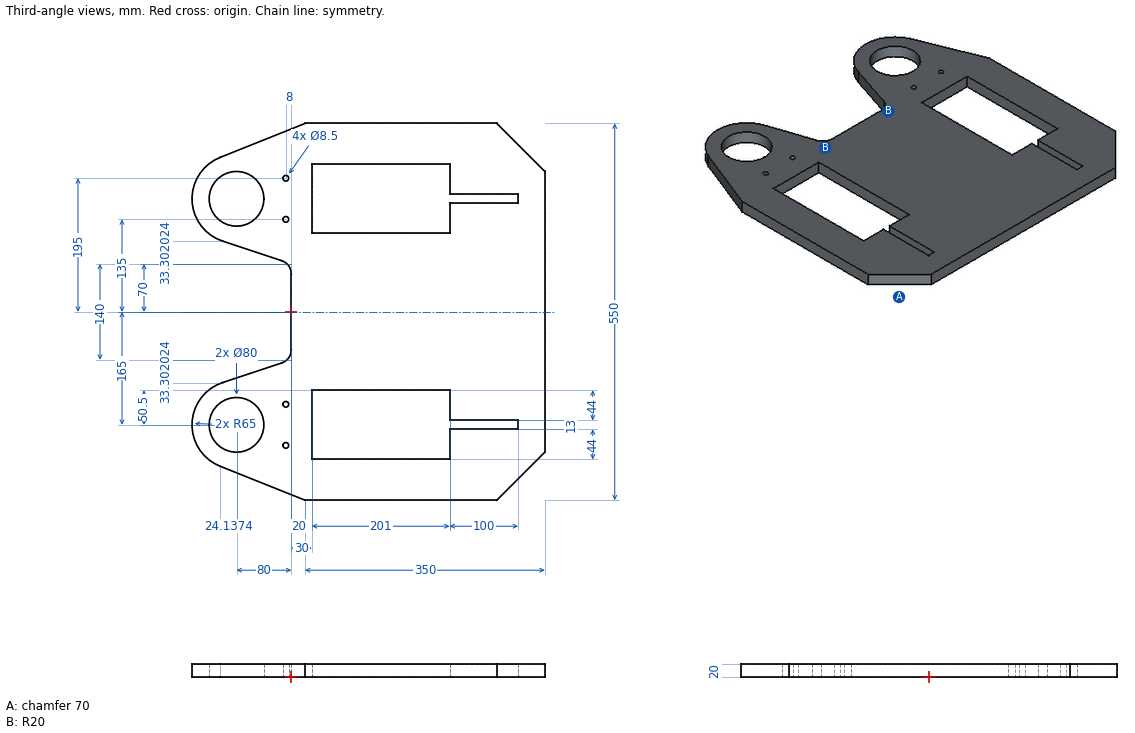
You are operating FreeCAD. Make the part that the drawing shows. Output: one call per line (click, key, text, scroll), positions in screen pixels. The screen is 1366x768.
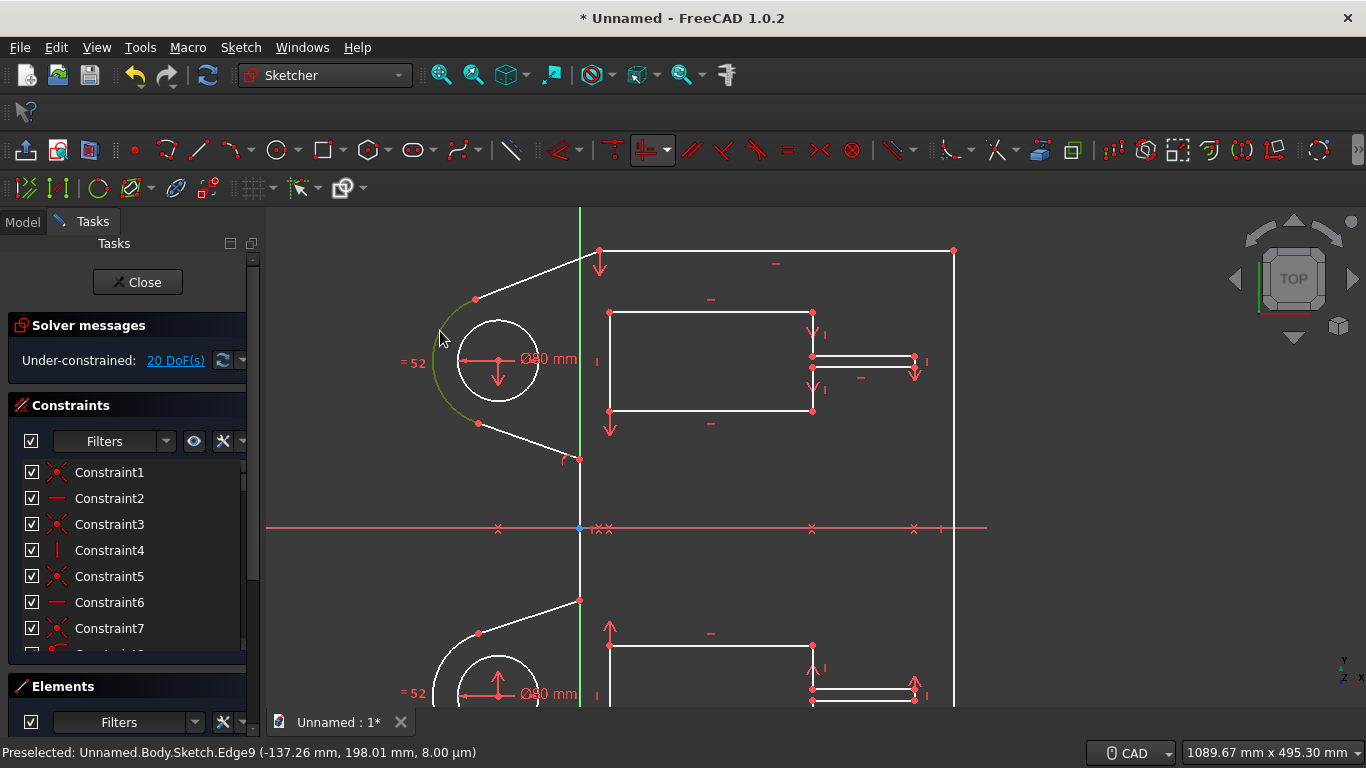
key(k)
key(r)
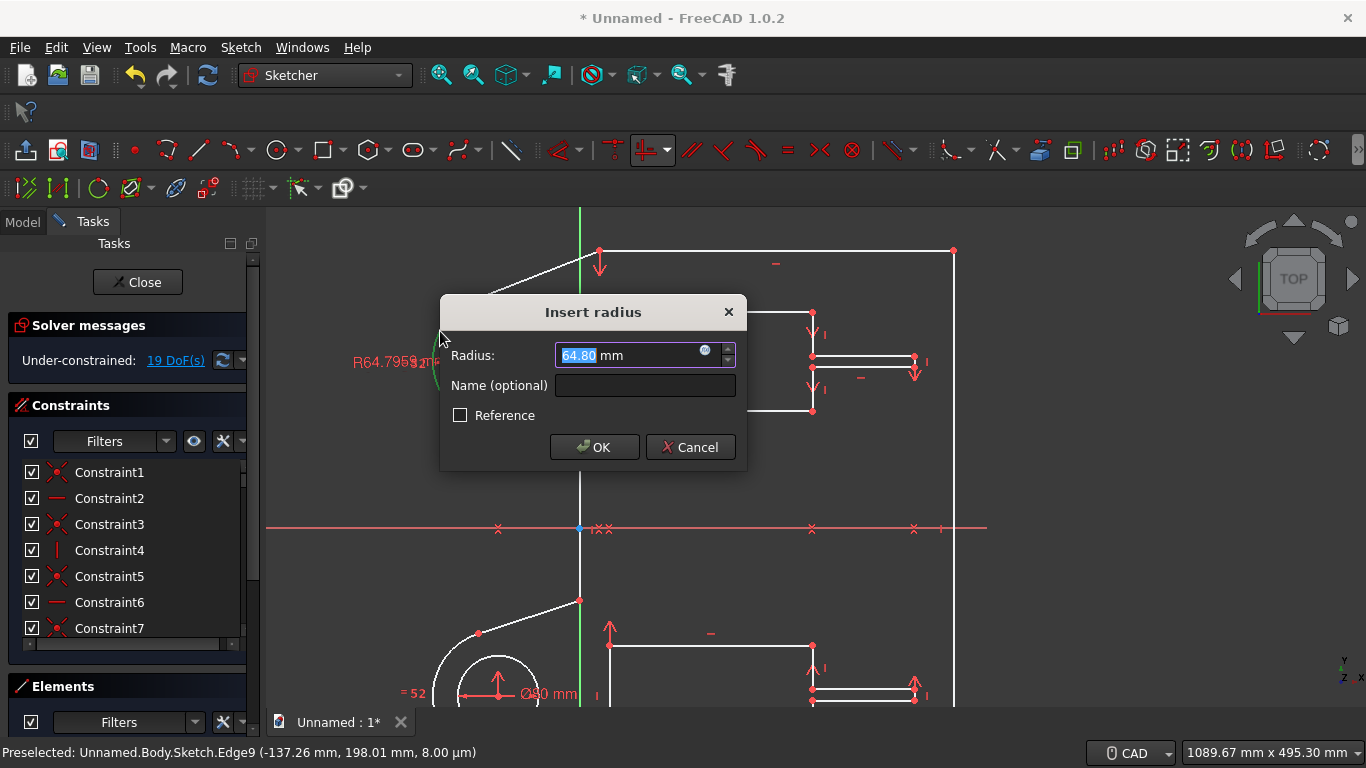
text(65)
key(Return)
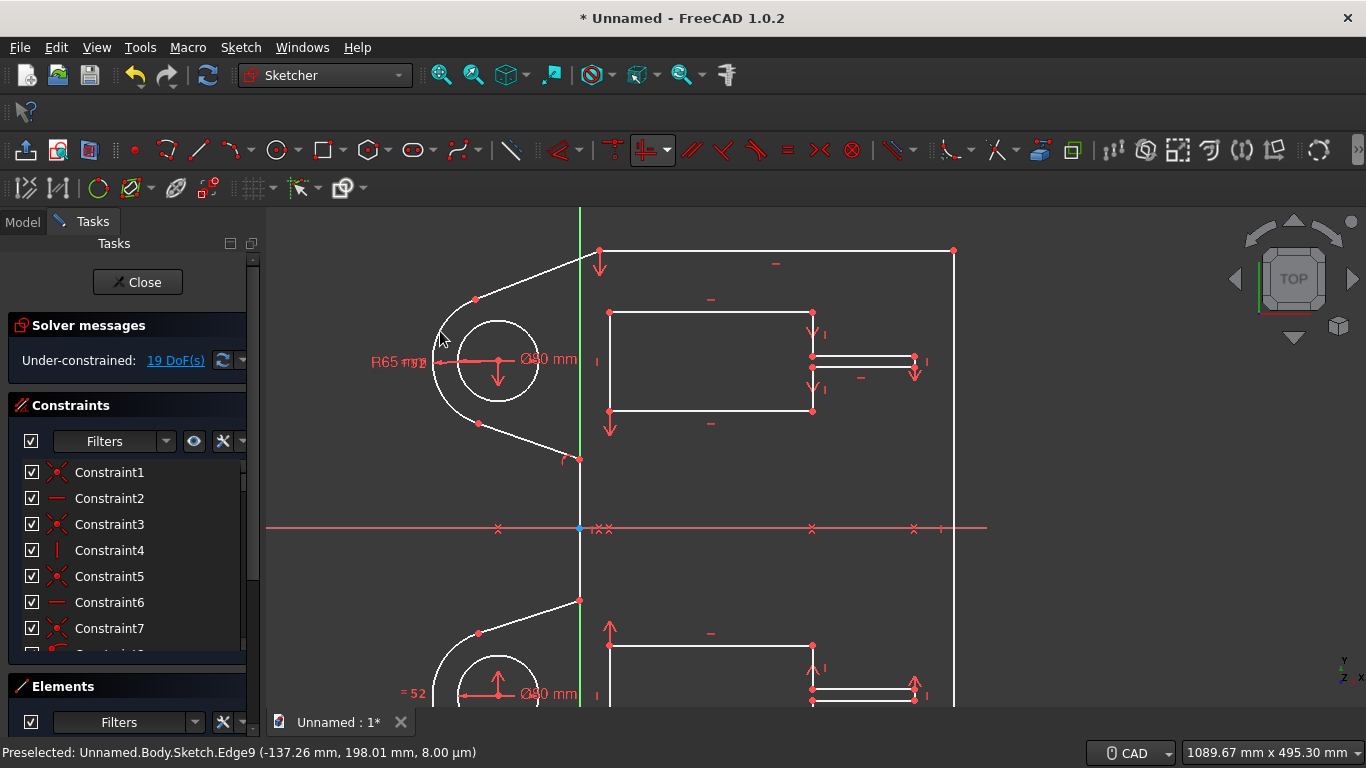
click(813, 676)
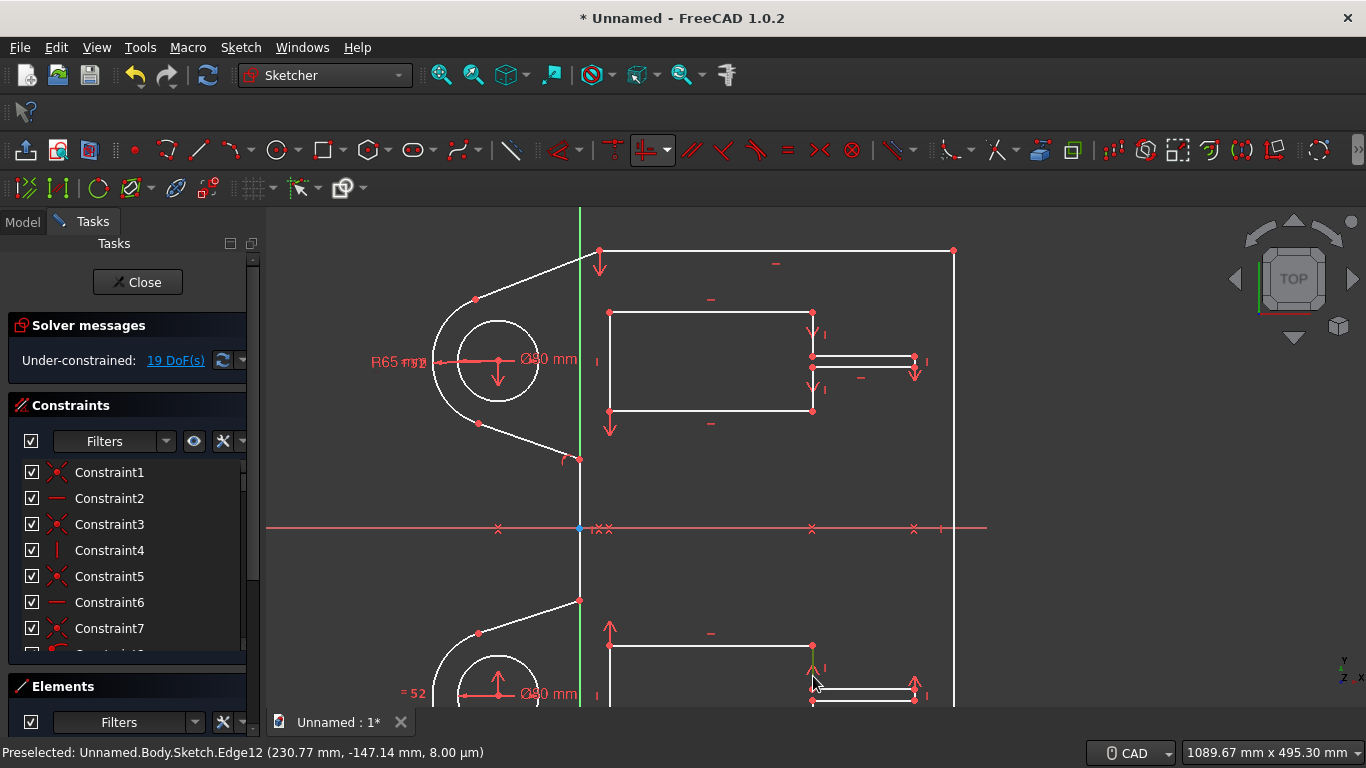
key(i)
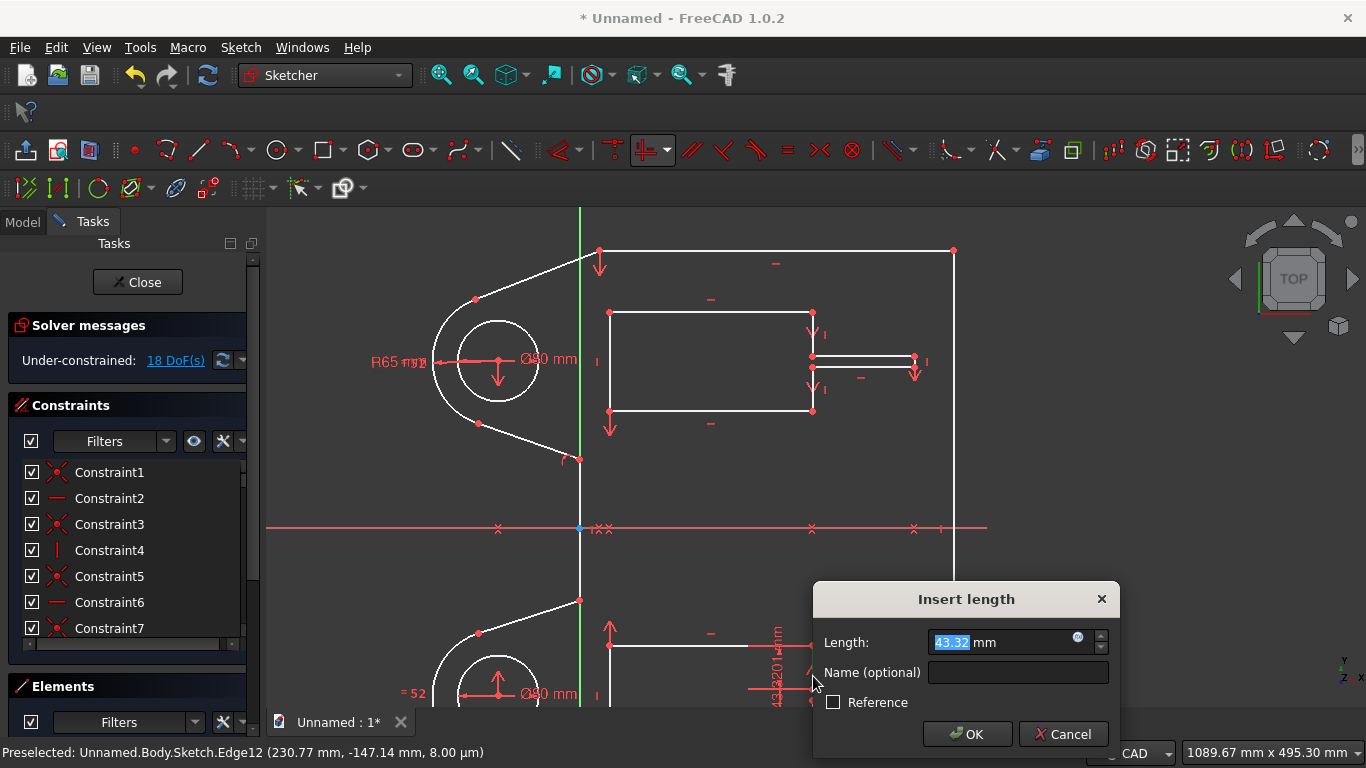
text(44)
key(Return)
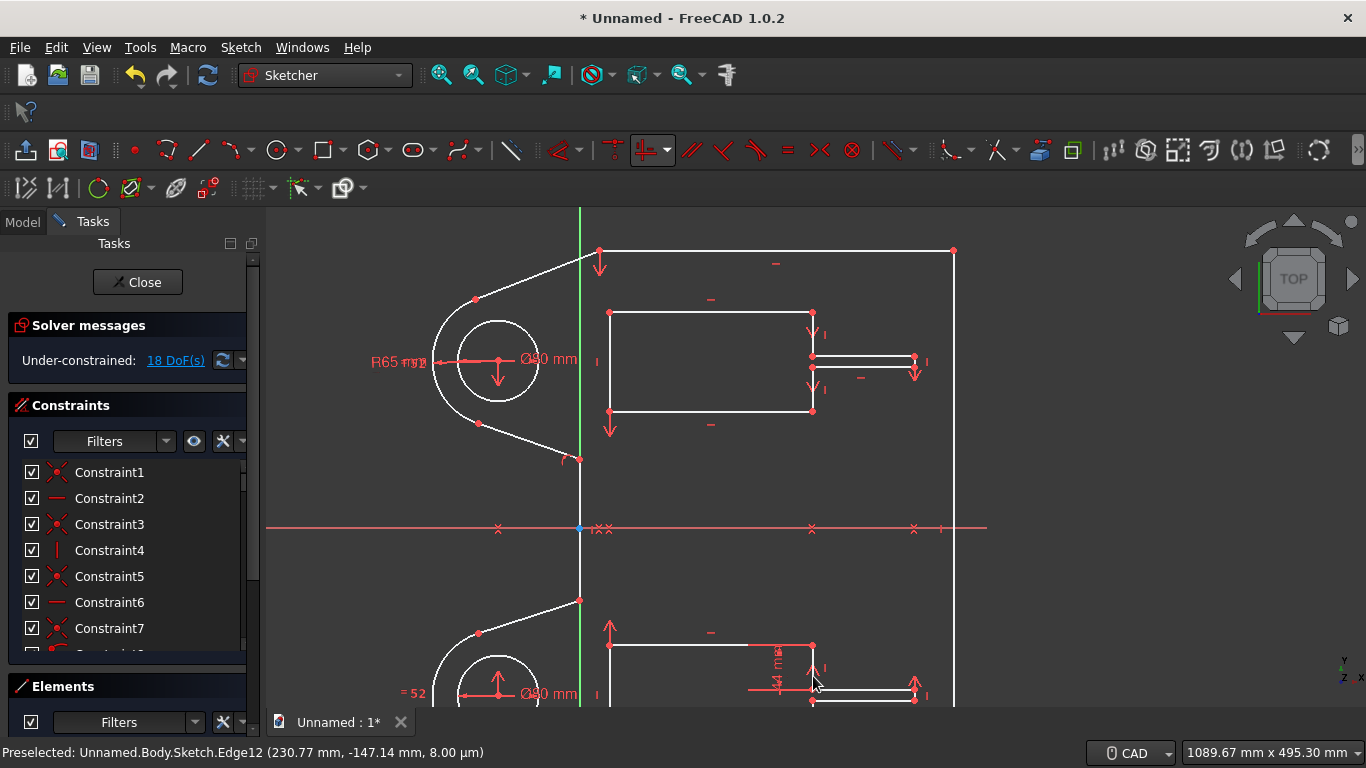
scroll(813, 370, down, 3)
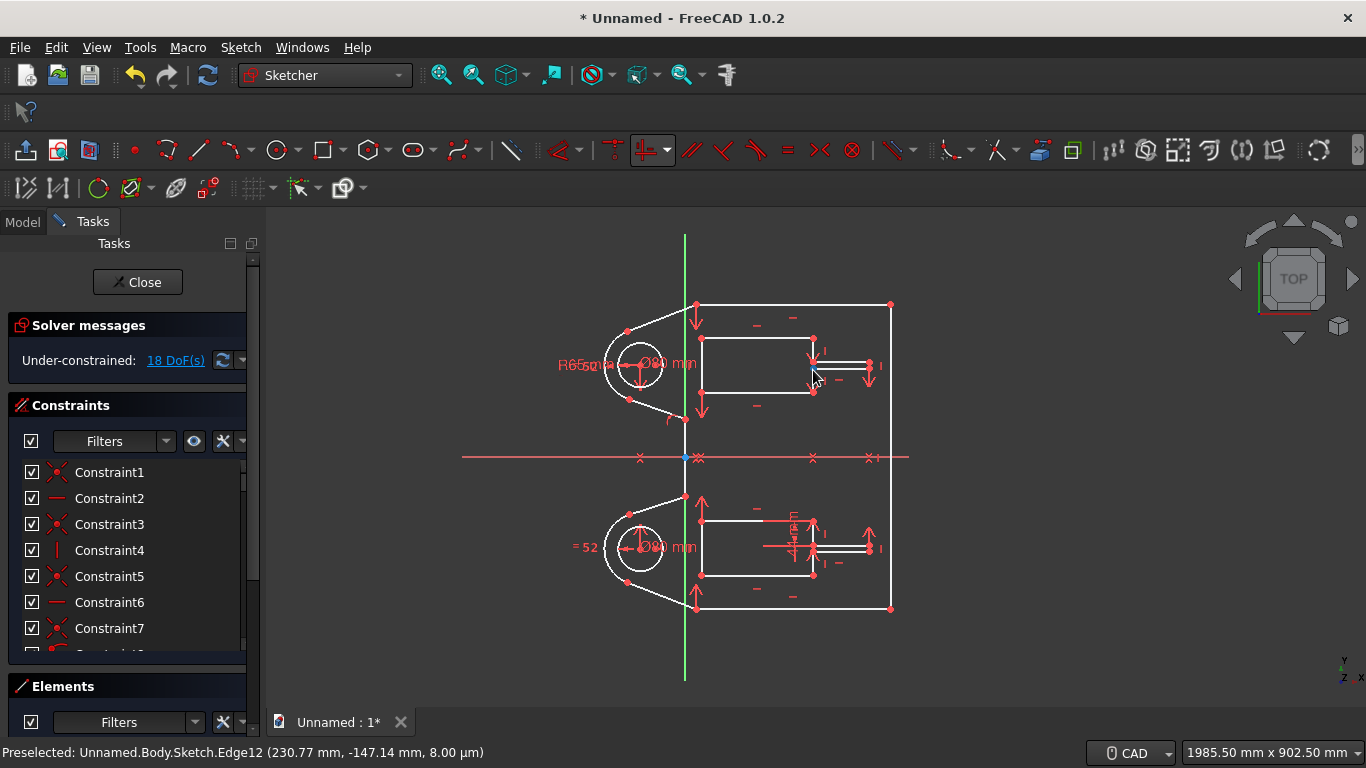
scroll(869, 549, up, 9)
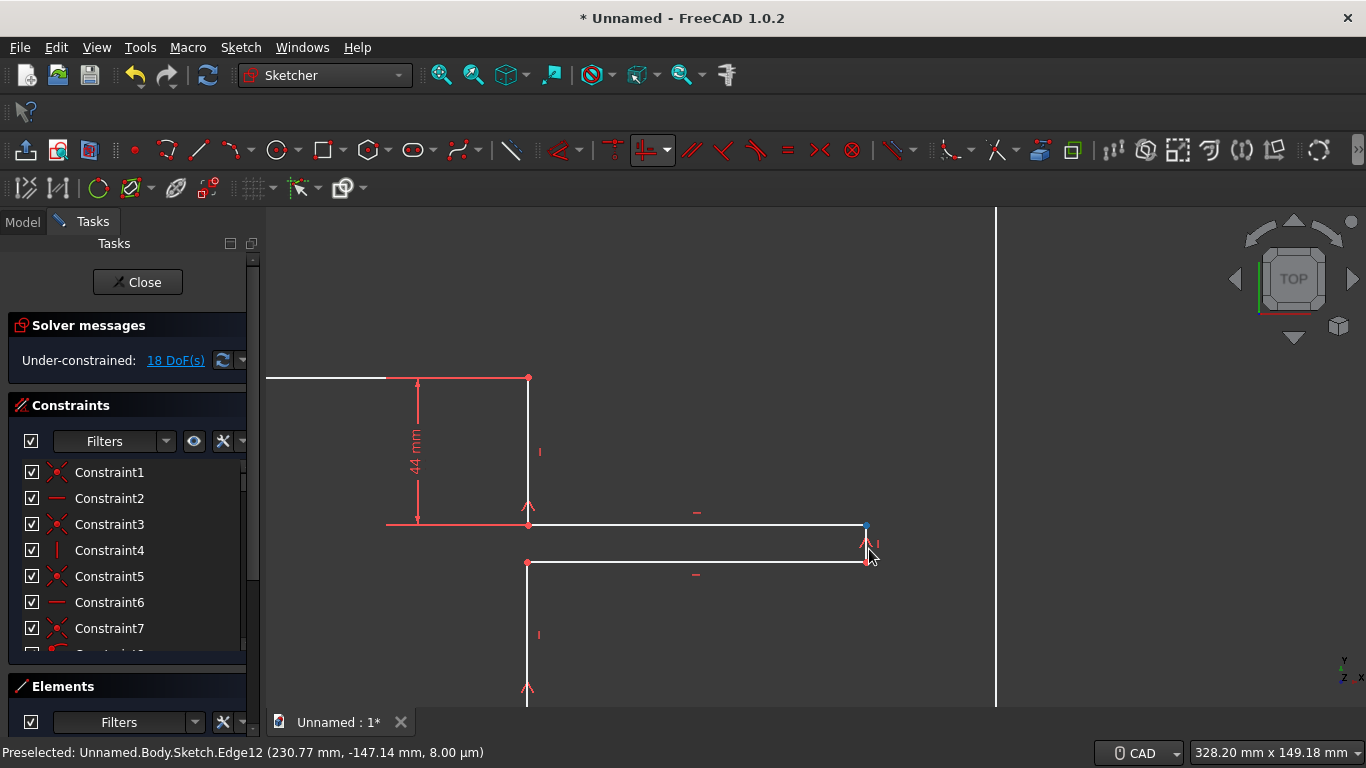
click(866, 544)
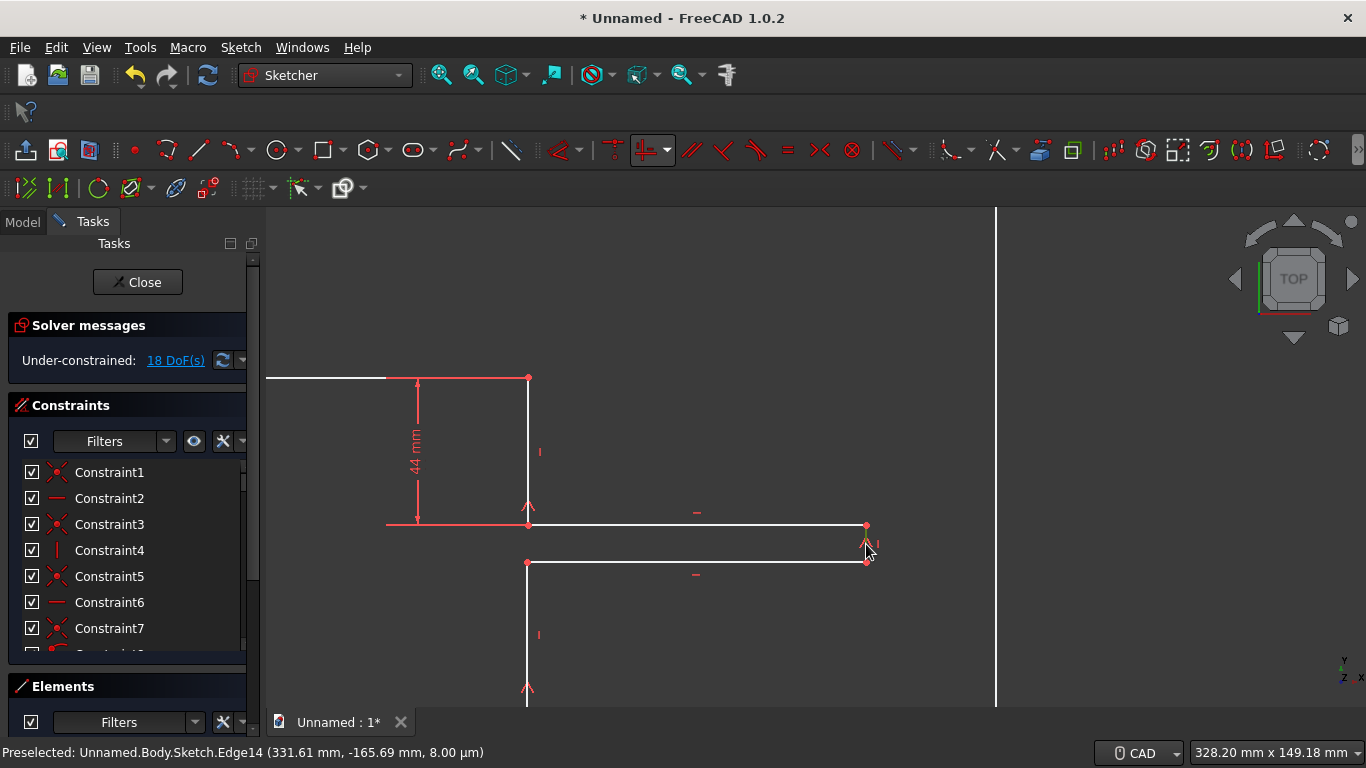
key(i)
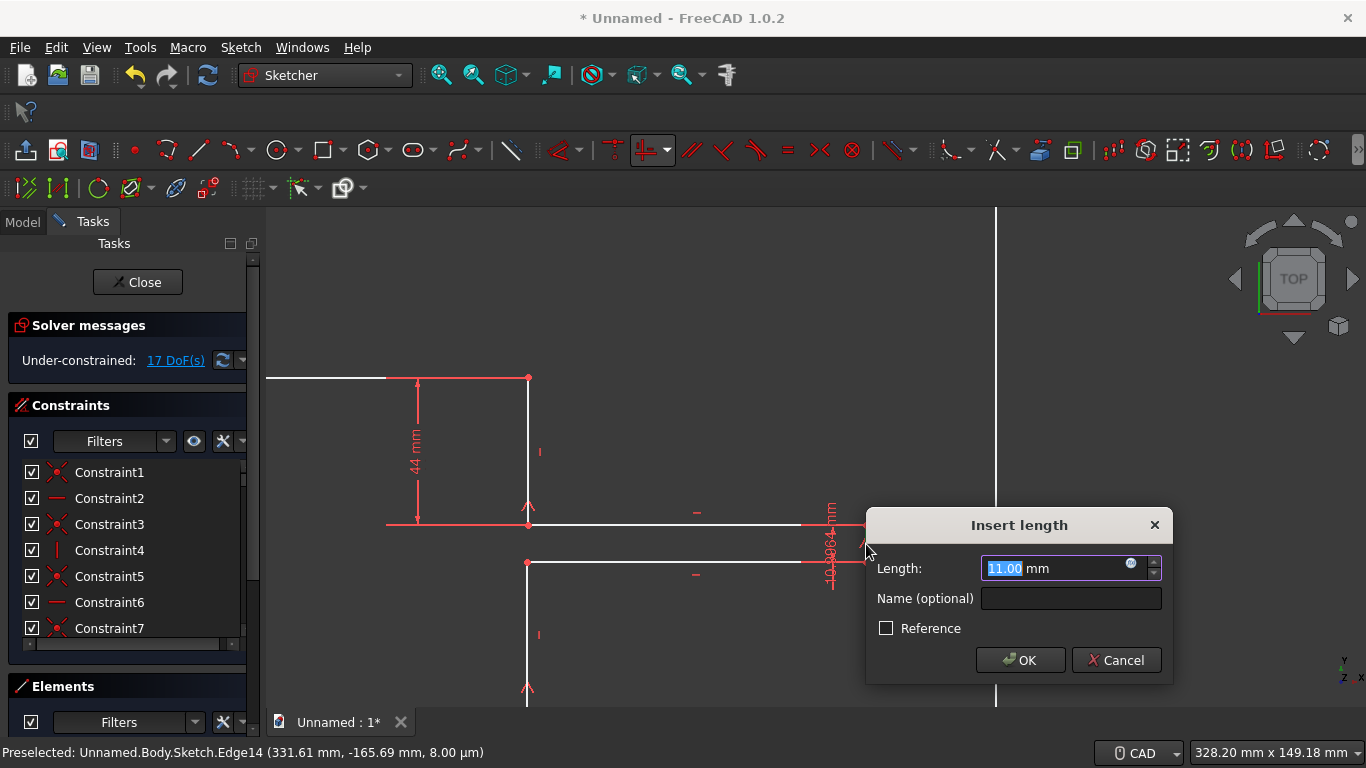
text(13)
key(Return)